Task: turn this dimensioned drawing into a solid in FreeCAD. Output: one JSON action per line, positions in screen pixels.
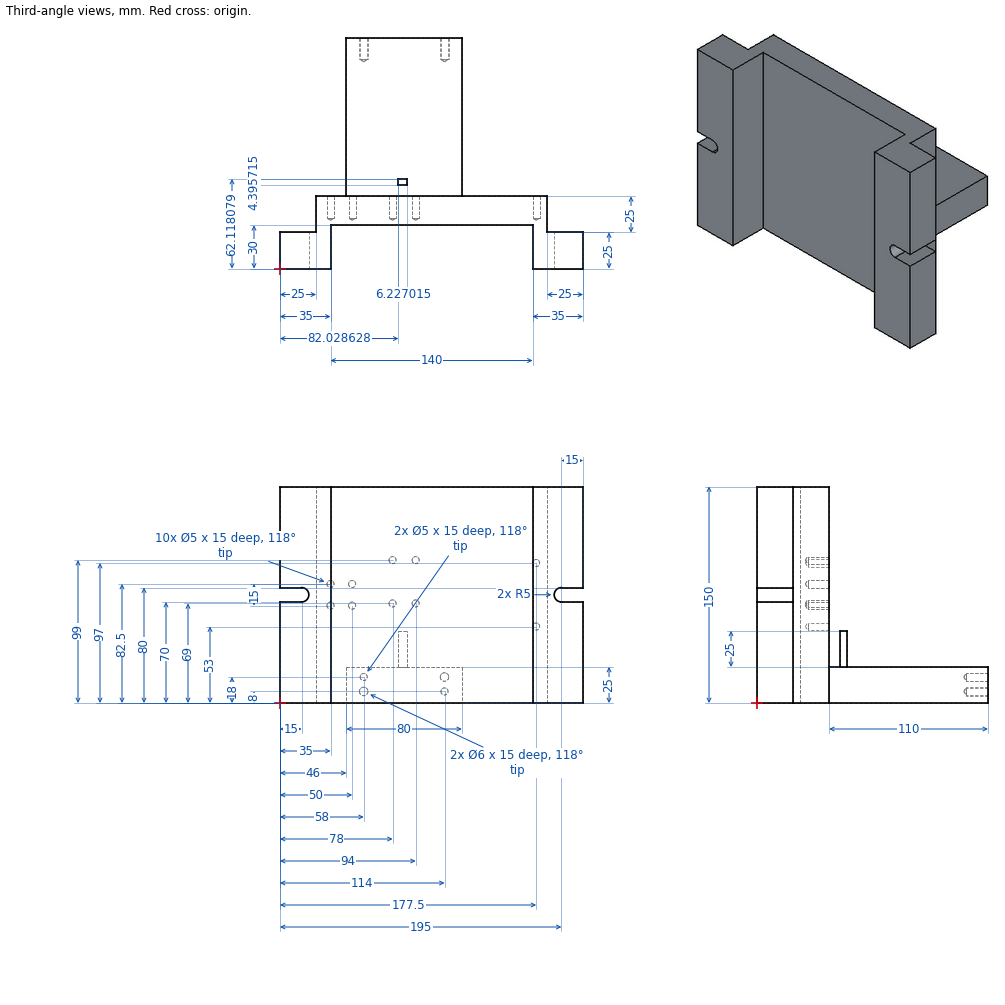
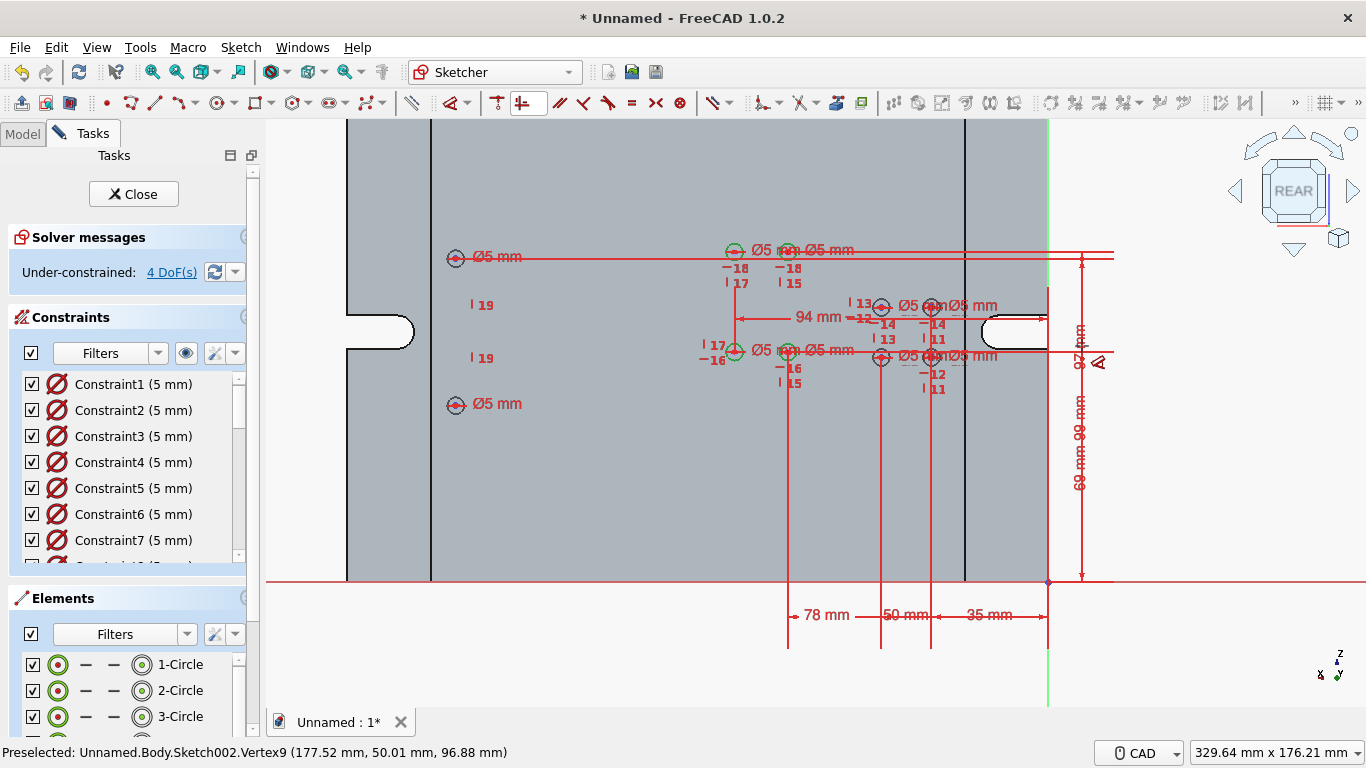
{"action": "left_click", "coordinate": [456, 406]}
{"action": "left_click", "coordinate": [1082, 494]}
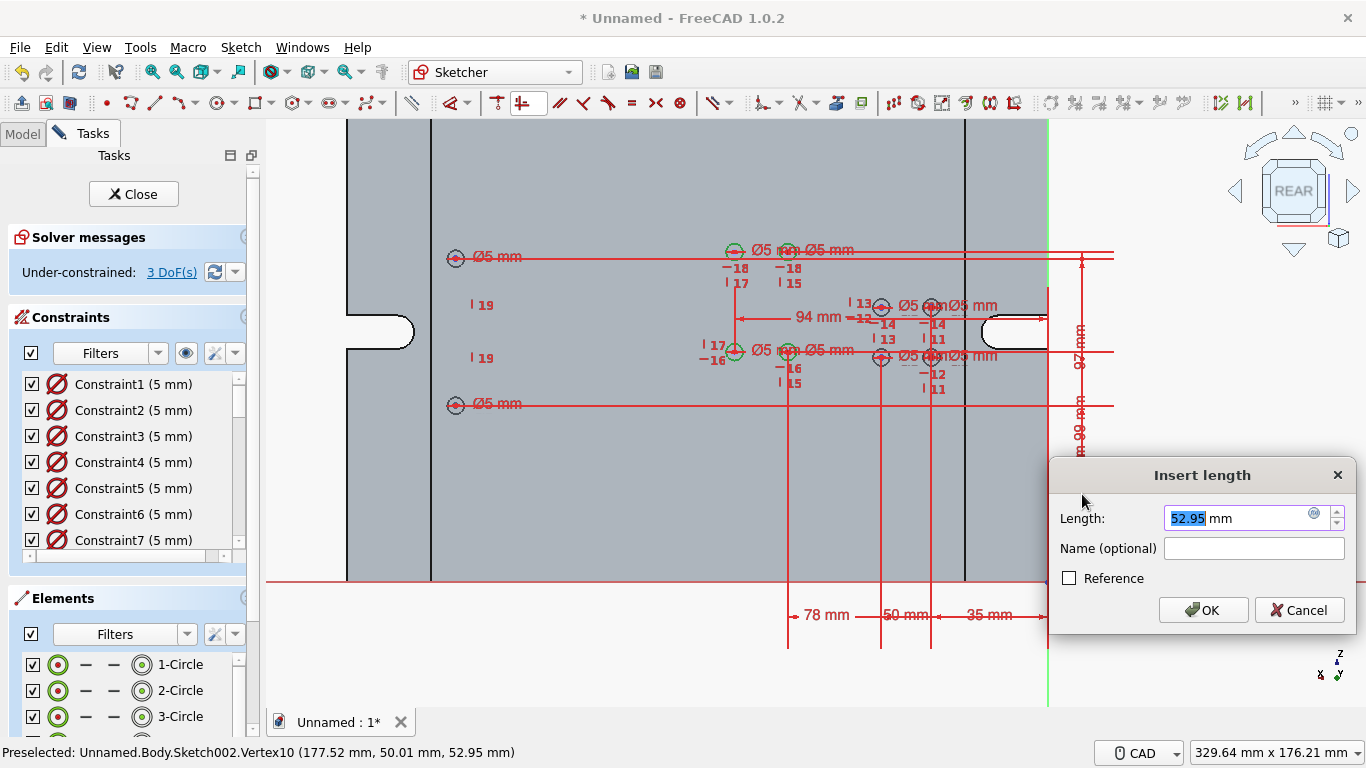
{"action": "type", "text": "53"}
{"action": "key", "text": "Return"}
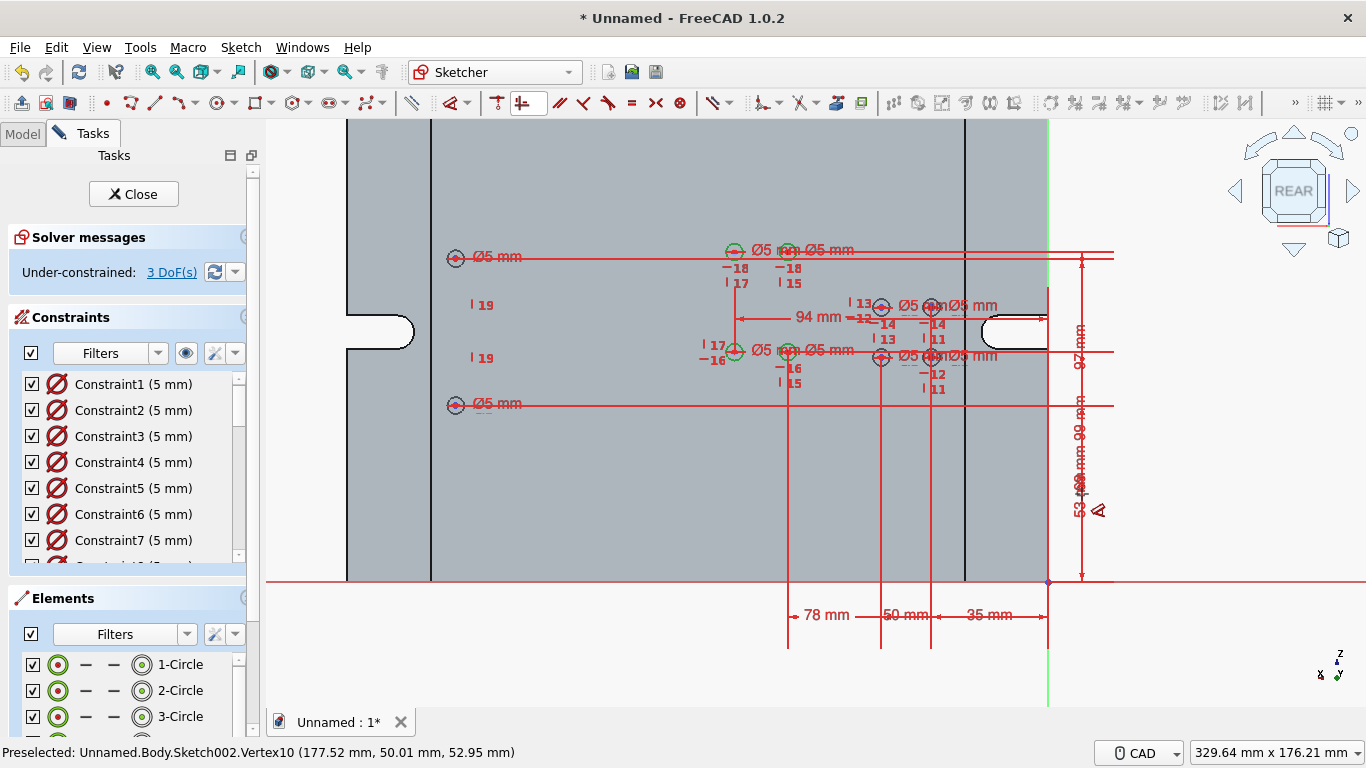
{"action": "left_click", "coordinate": [931, 308]}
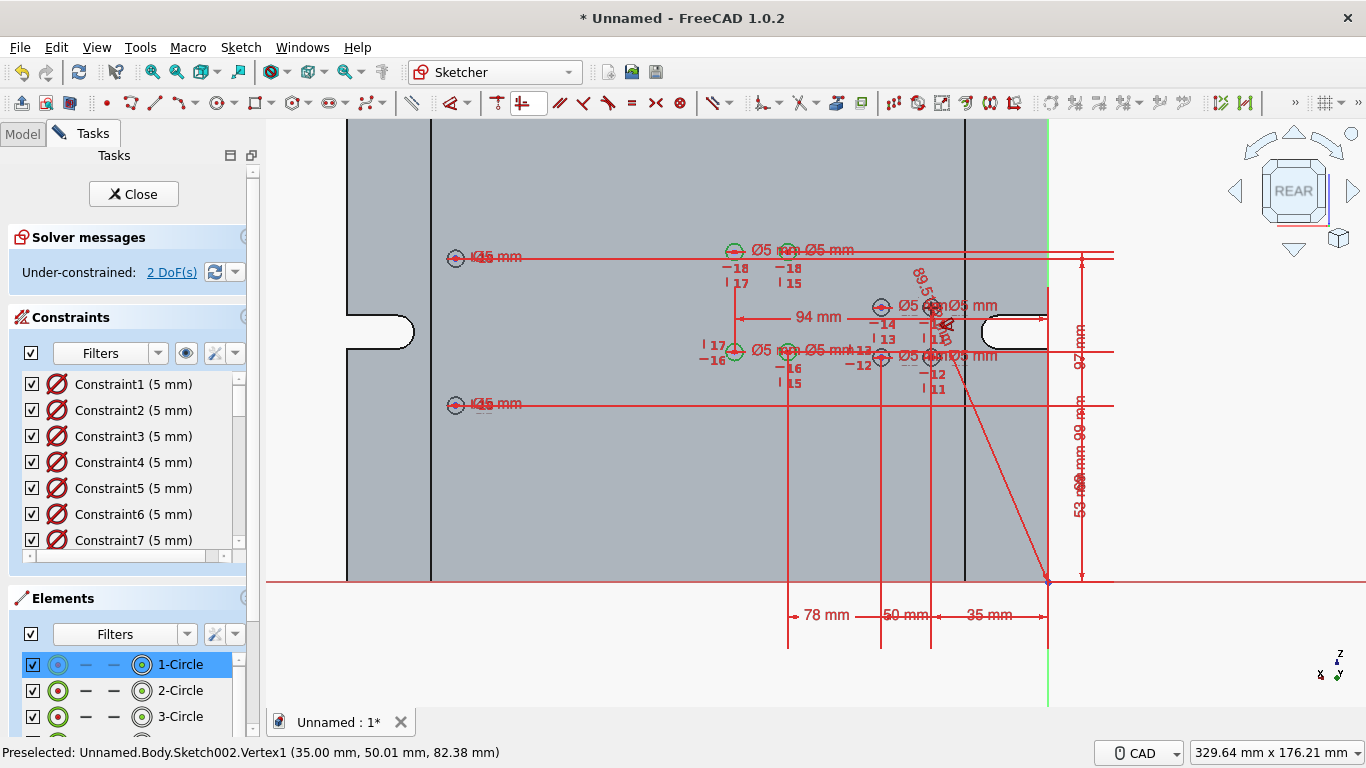
{"action": "left_click", "coordinate": [931, 358]}
{"action": "left_click", "coordinate": [965, 333]}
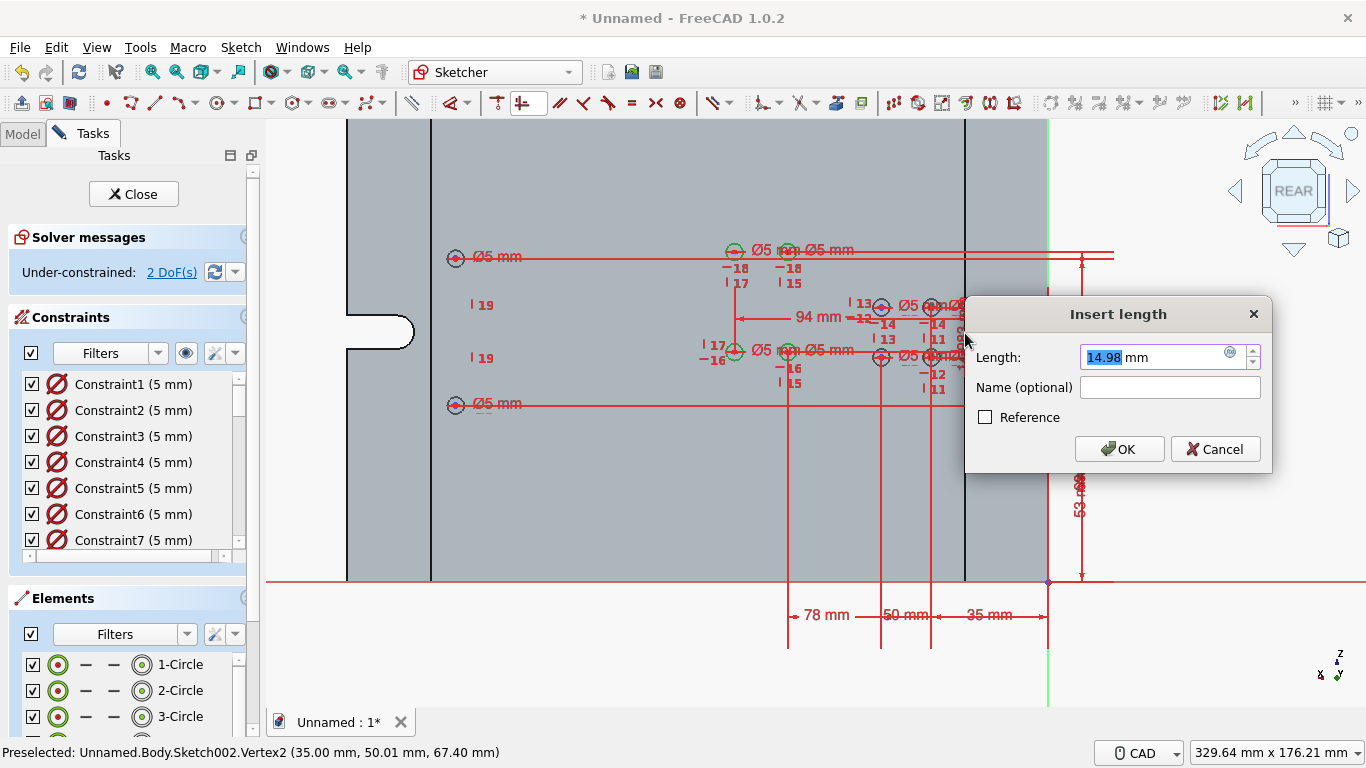
{"action": "type", "text": "15"}
{"action": "key", "text": "Return"}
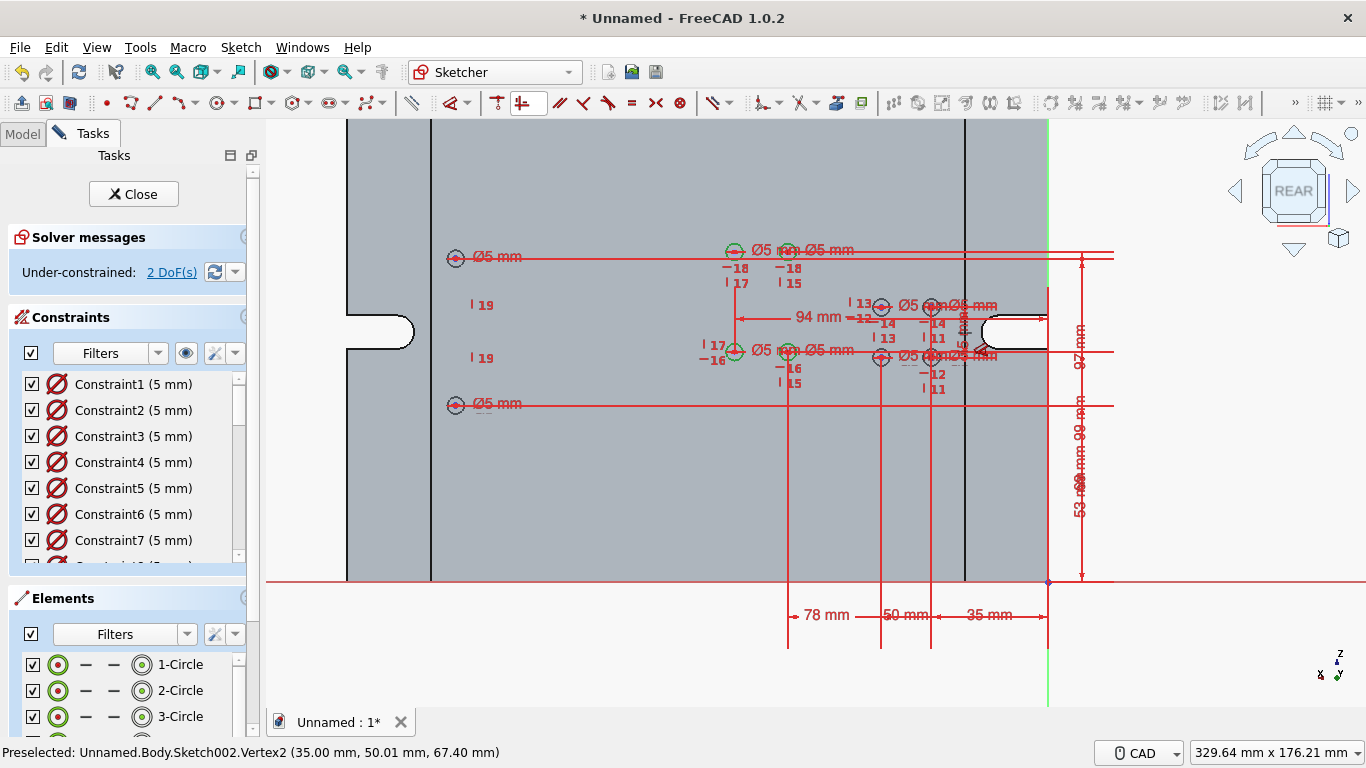
{"action": "left_click", "coordinate": [931, 307]}
{"action": "left_click", "coordinate": [1082, 445]}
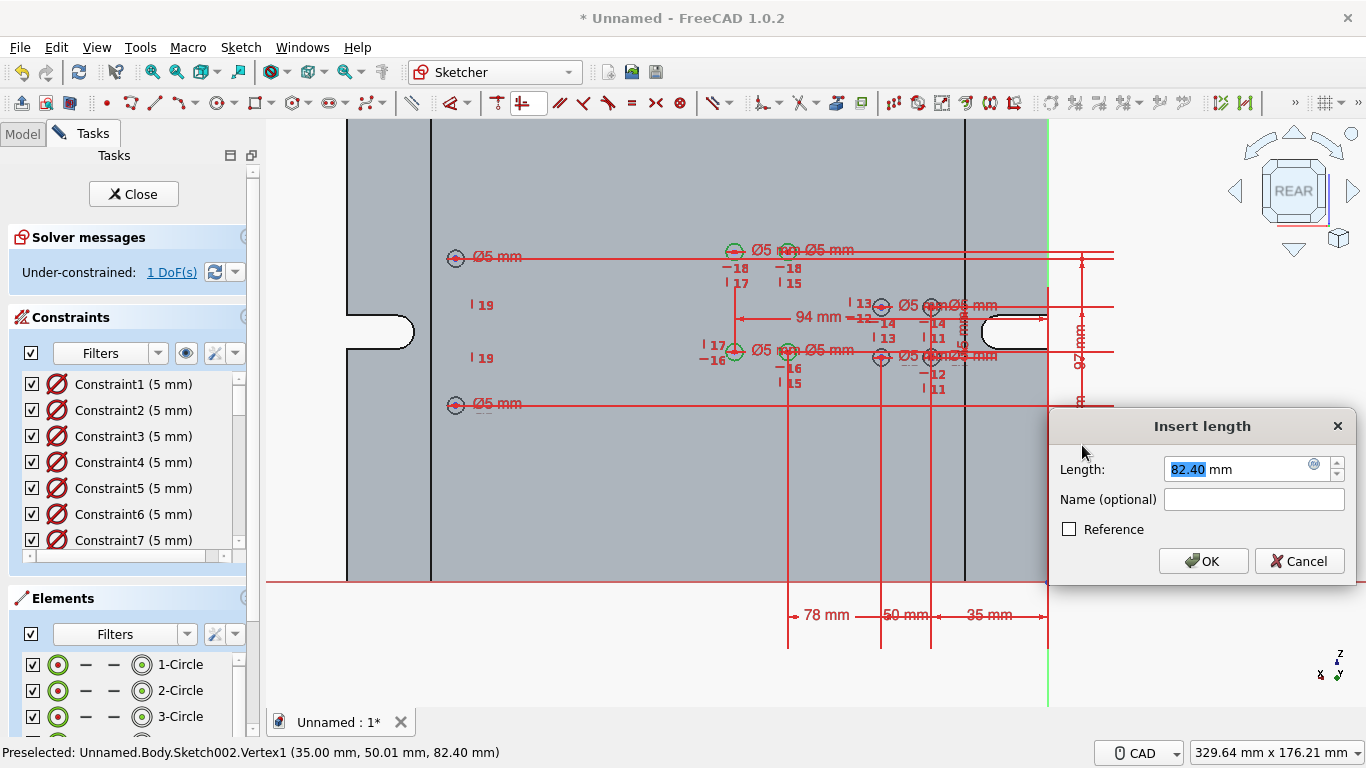
{"action": "type", "text": "82.5"}
{"action": "key", "text": "Return"}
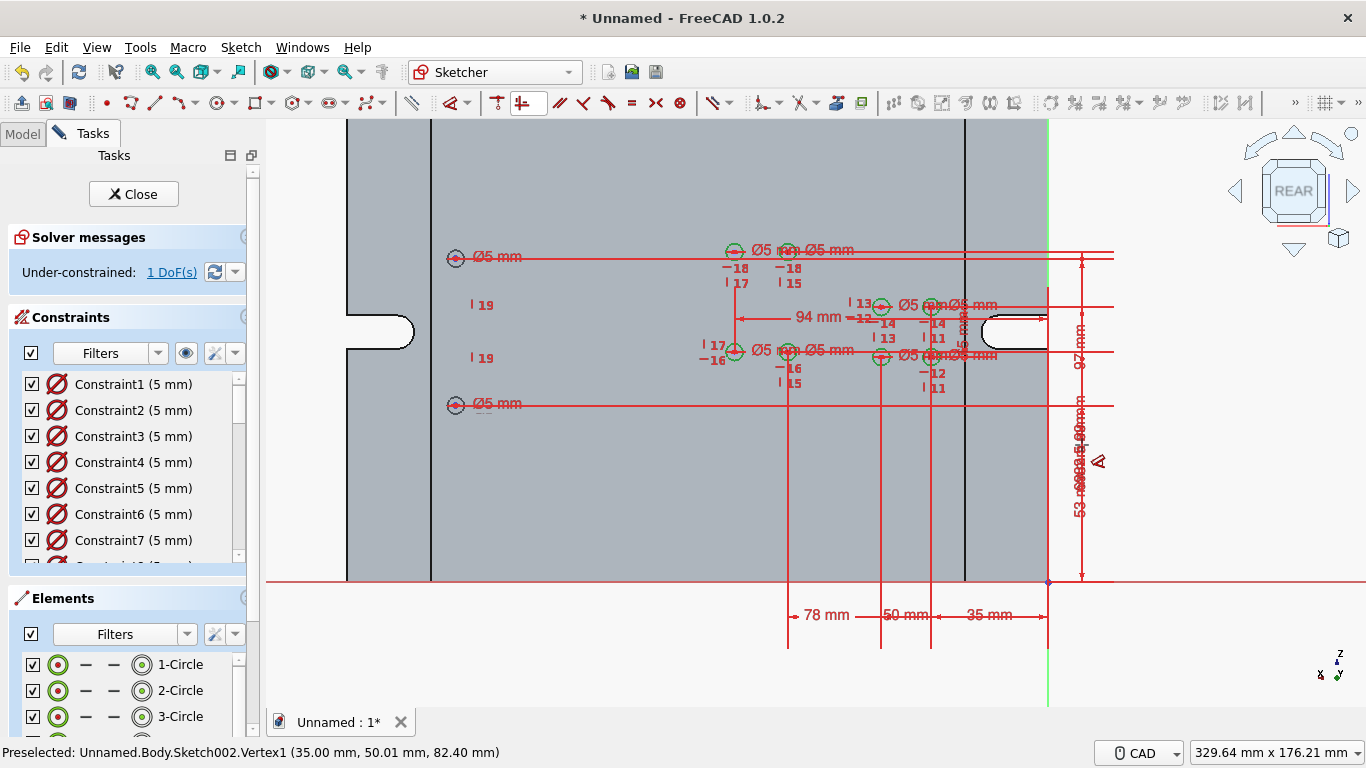
{"action": "left_click", "coordinate": [456, 259]}
{"action": "left_click", "coordinate": [752, 616]}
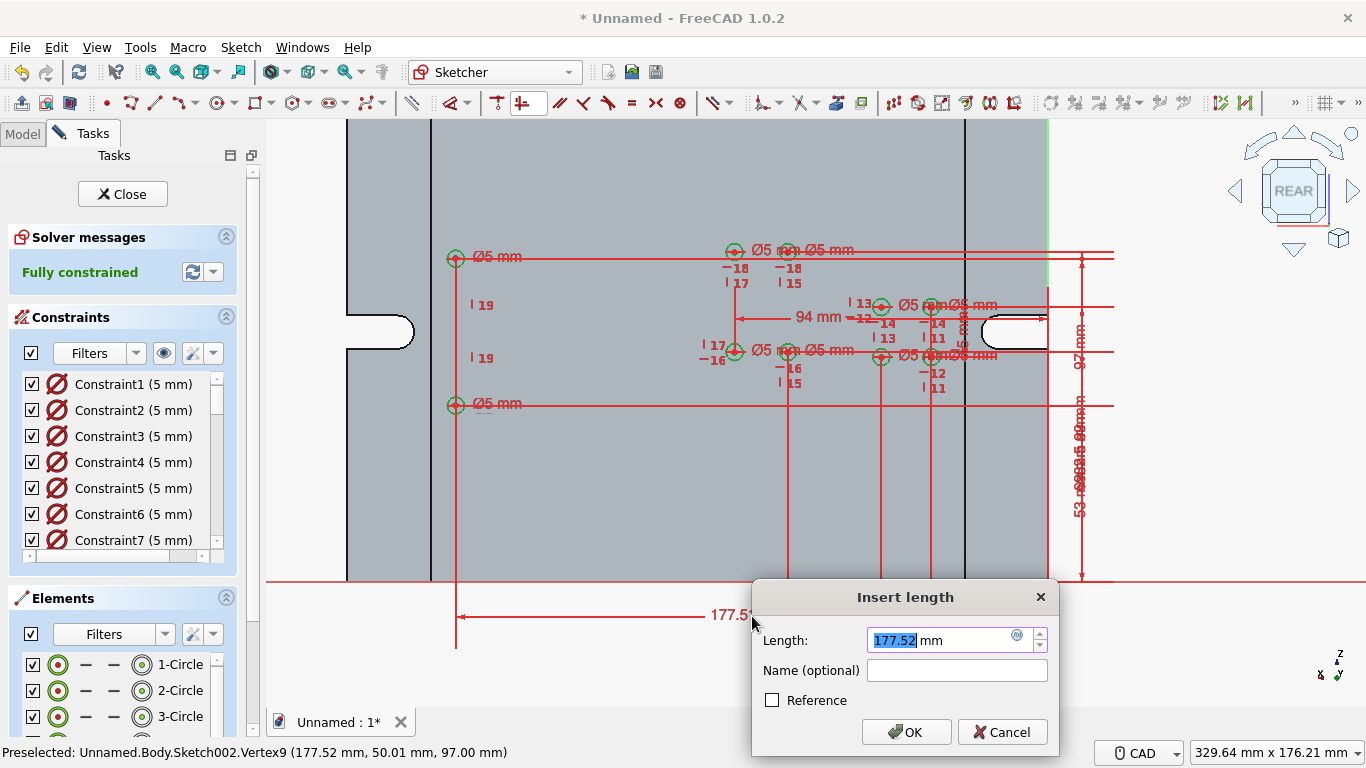
{"action": "type", "text": "177.5"}
{"action": "key", "text": "Return"}
{"action": "key", "text": "Escape"}